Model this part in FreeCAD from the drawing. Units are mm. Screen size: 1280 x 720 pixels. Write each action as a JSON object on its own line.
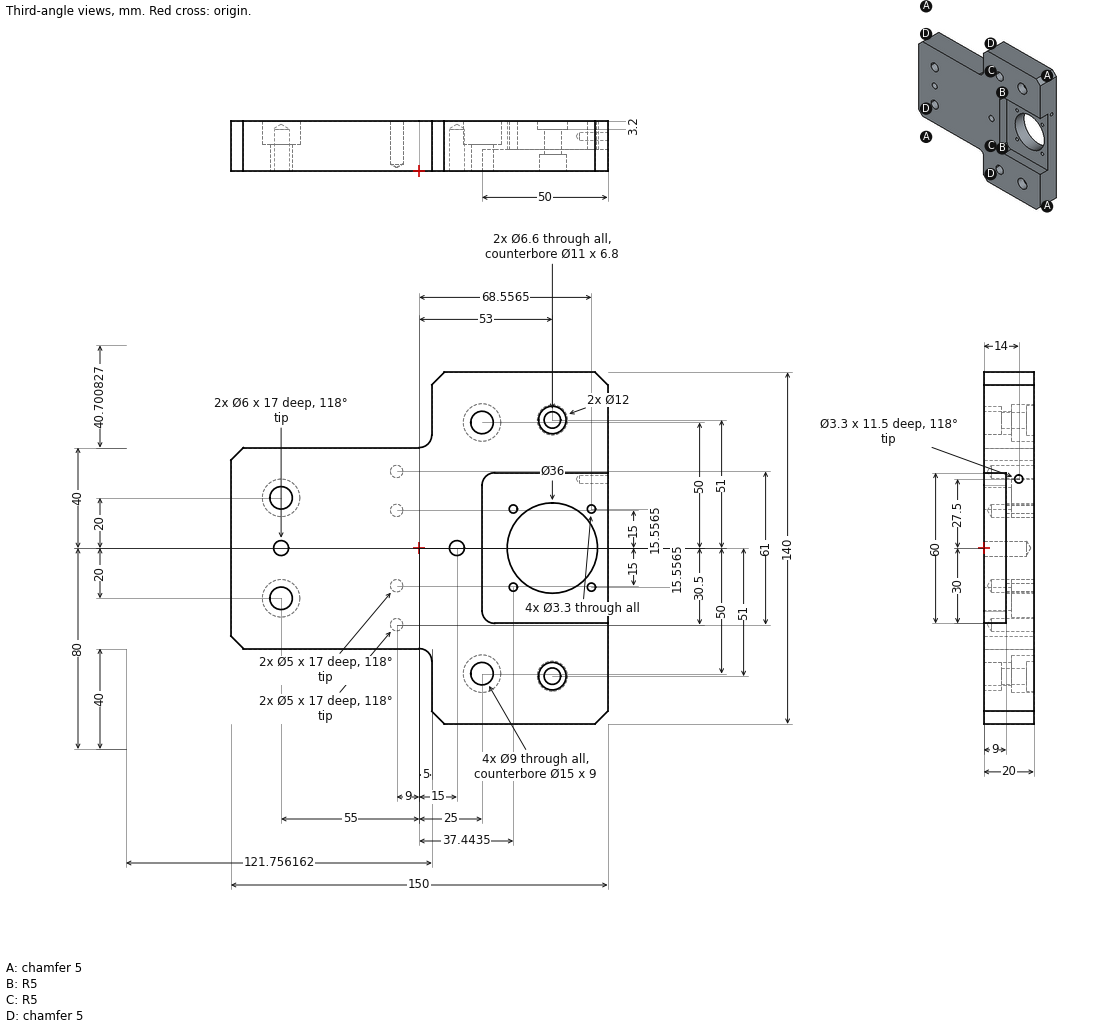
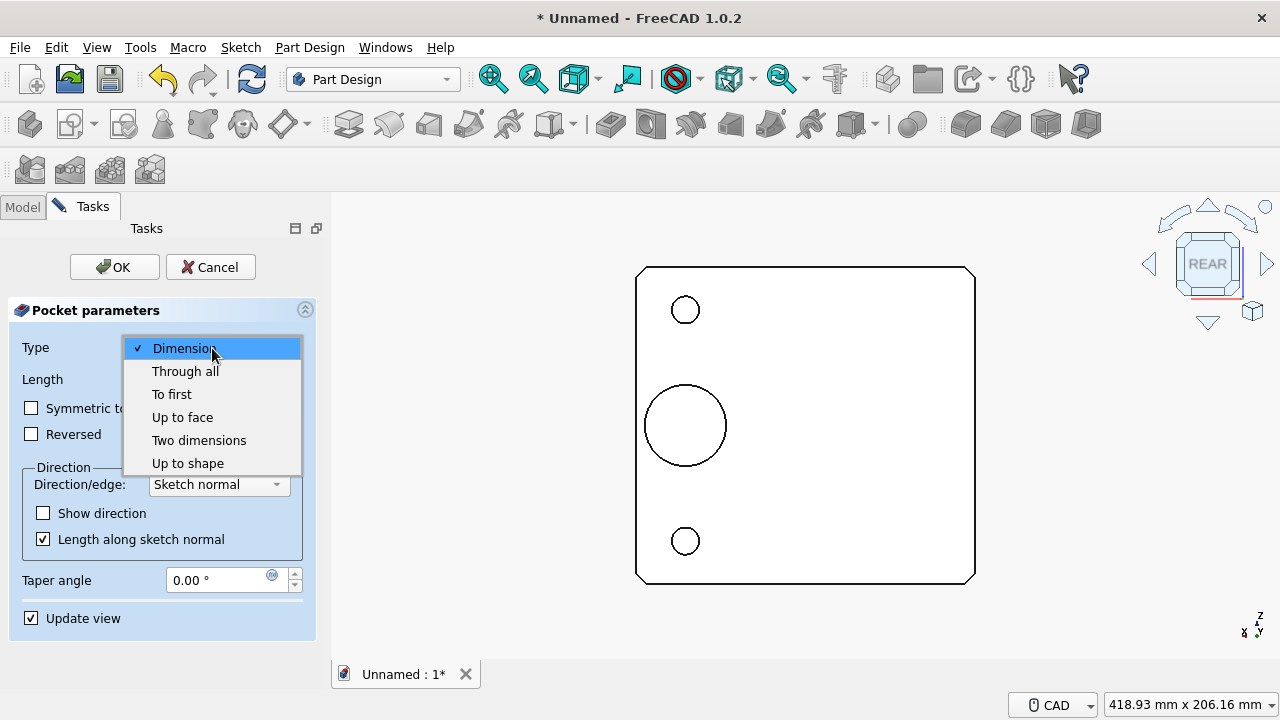
{"action": "left_click", "coordinate": [212, 372]}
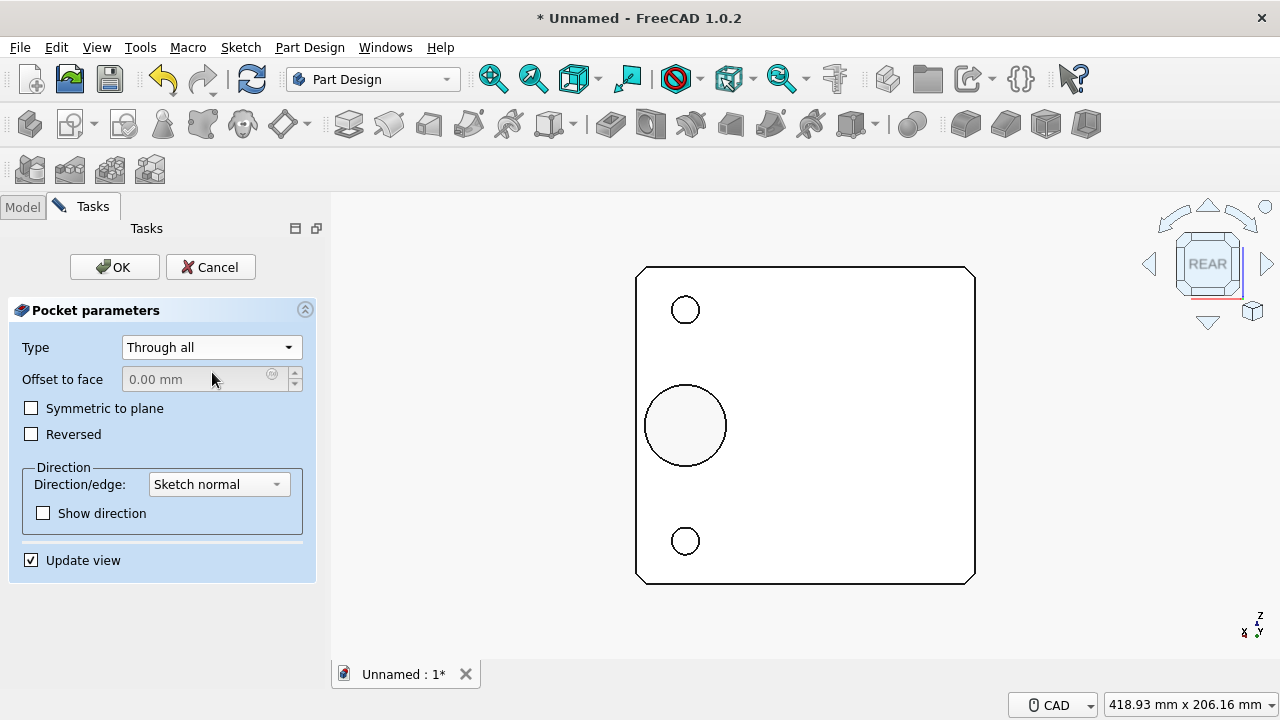
{"action": "left_click", "coordinate": [115, 267]}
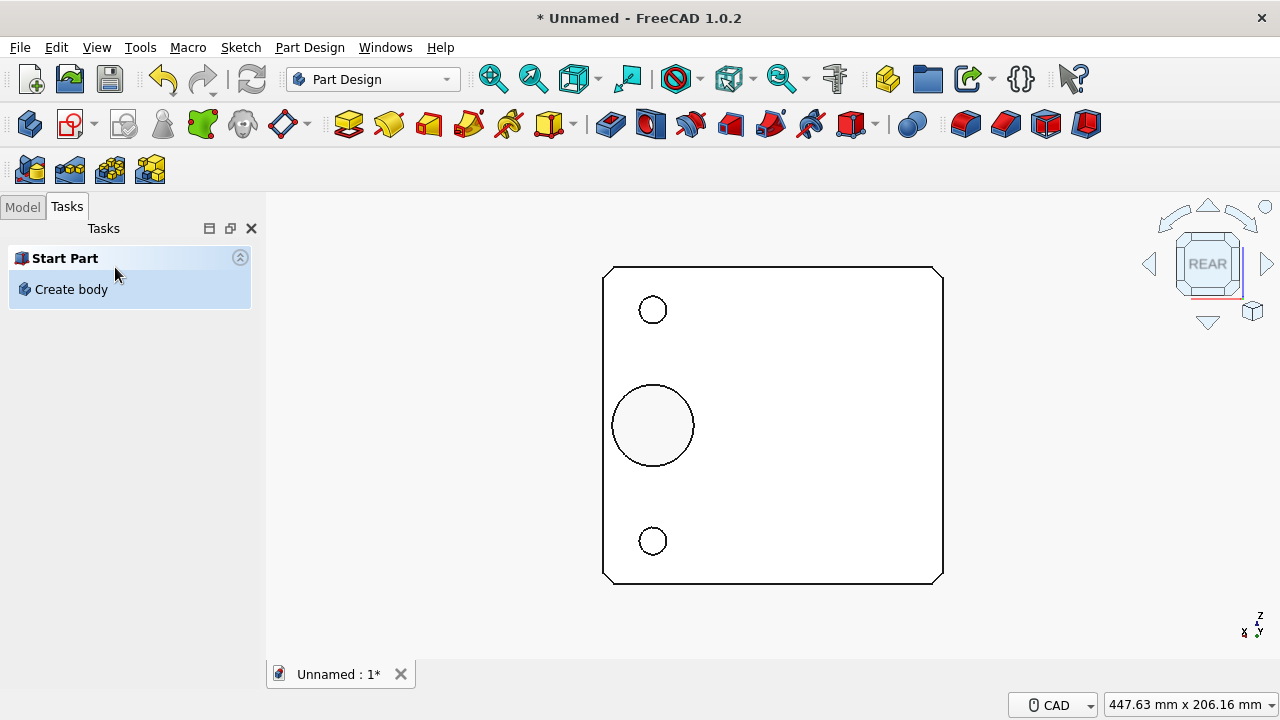
{"action": "left_click", "coordinate": [822, 424]}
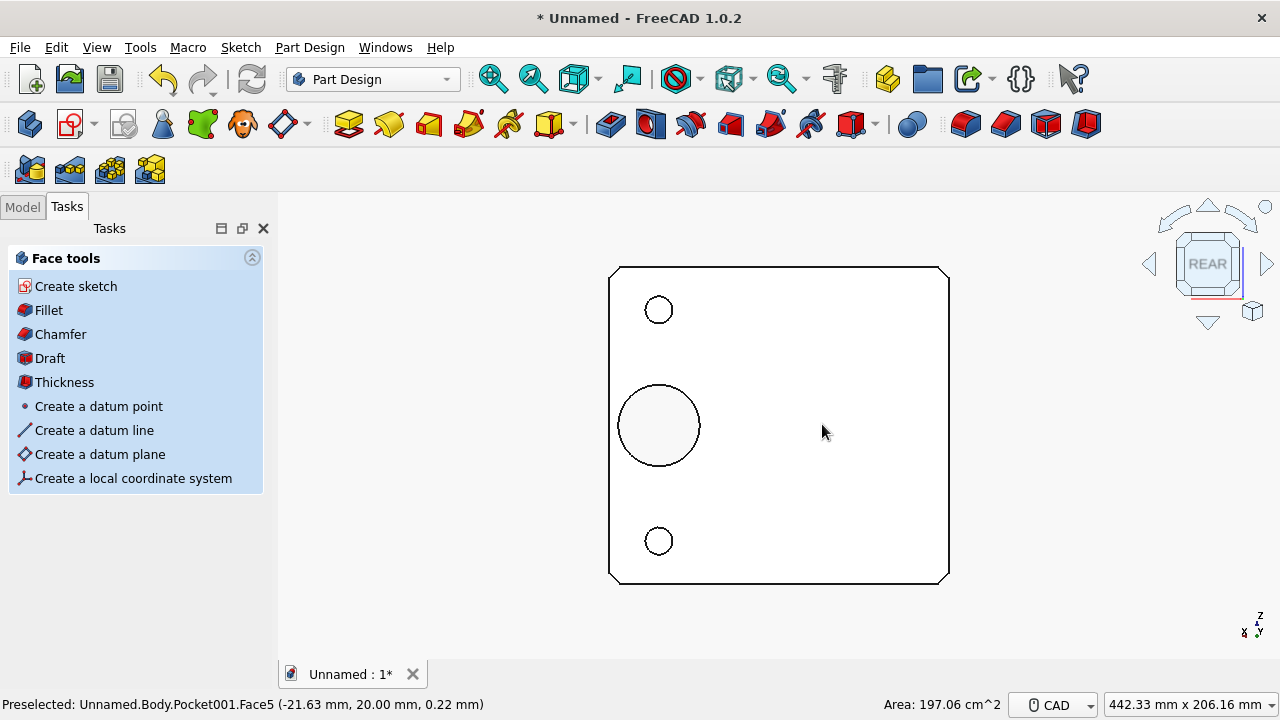
{"action": "left_click", "coordinate": [70, 124]}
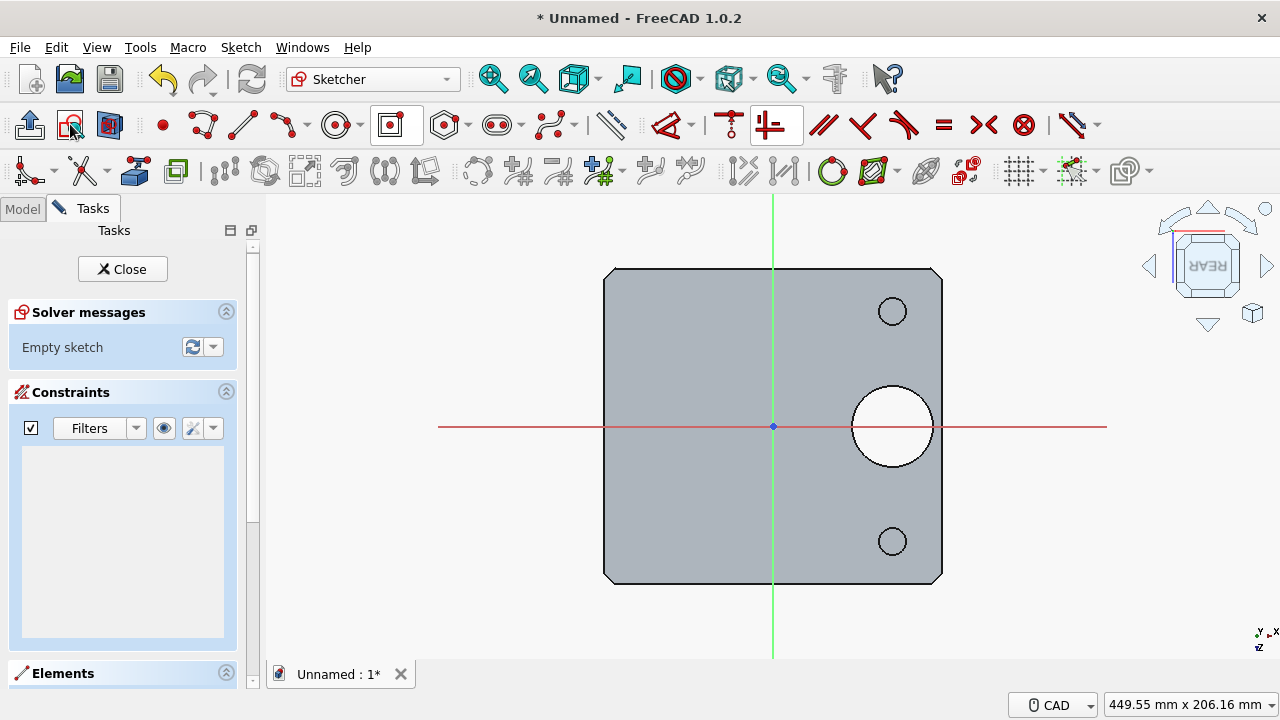
{"action": "scroll", "coordinate": [916, 426], "scroll_direction": "up", "scroll_amount": 6}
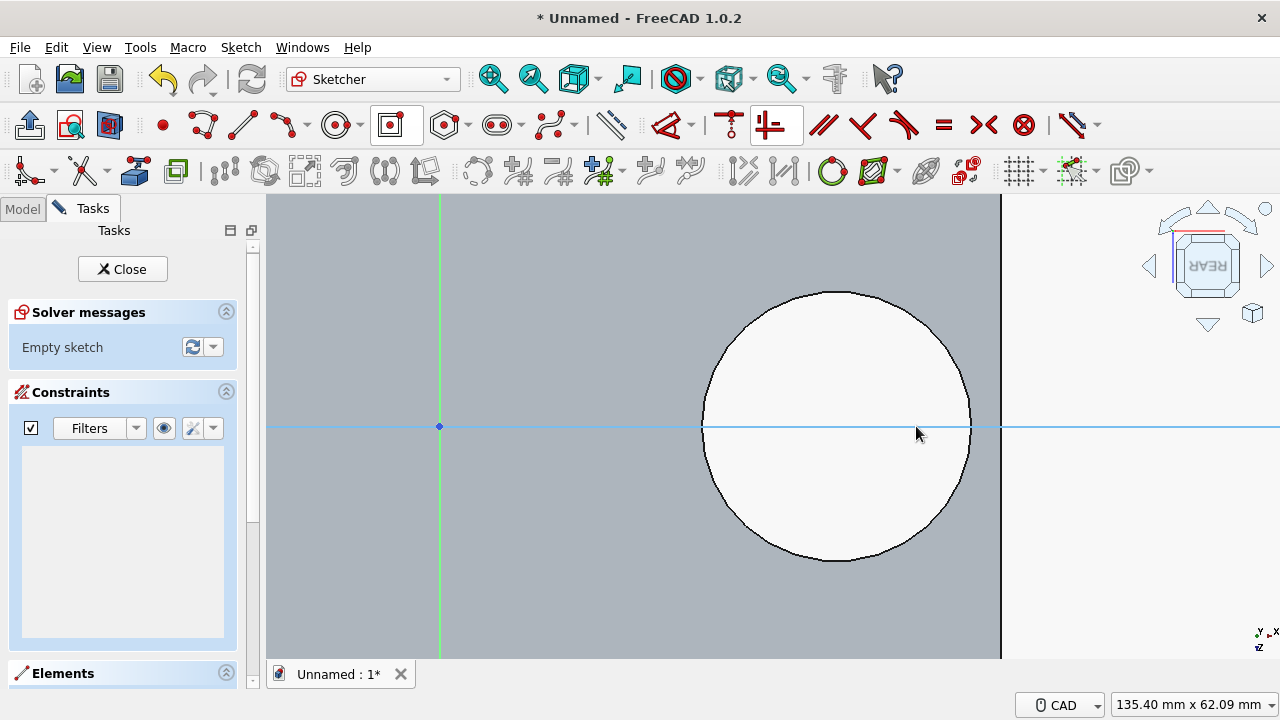
{"action": "left_click", "coordinate": [336, 126]}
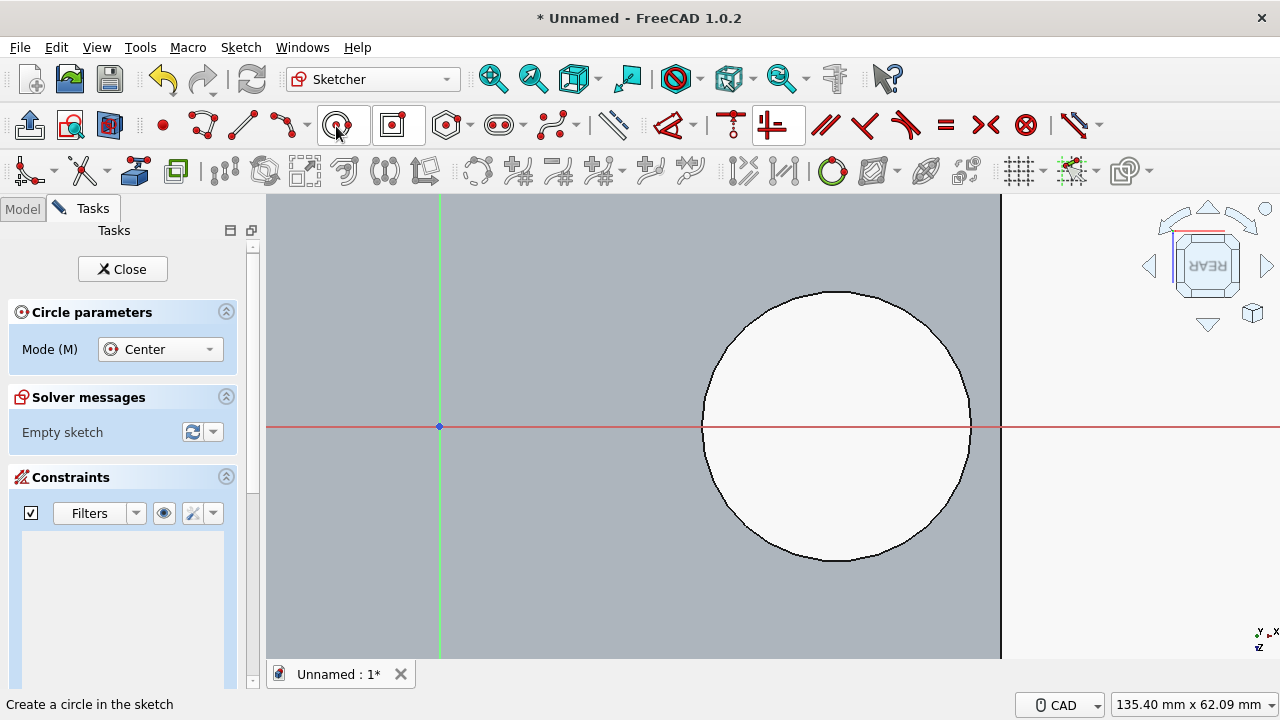
{"action": "scroll", "coordinate": [953, 543], "scroll_direction": "up", "scroll_amount": 4}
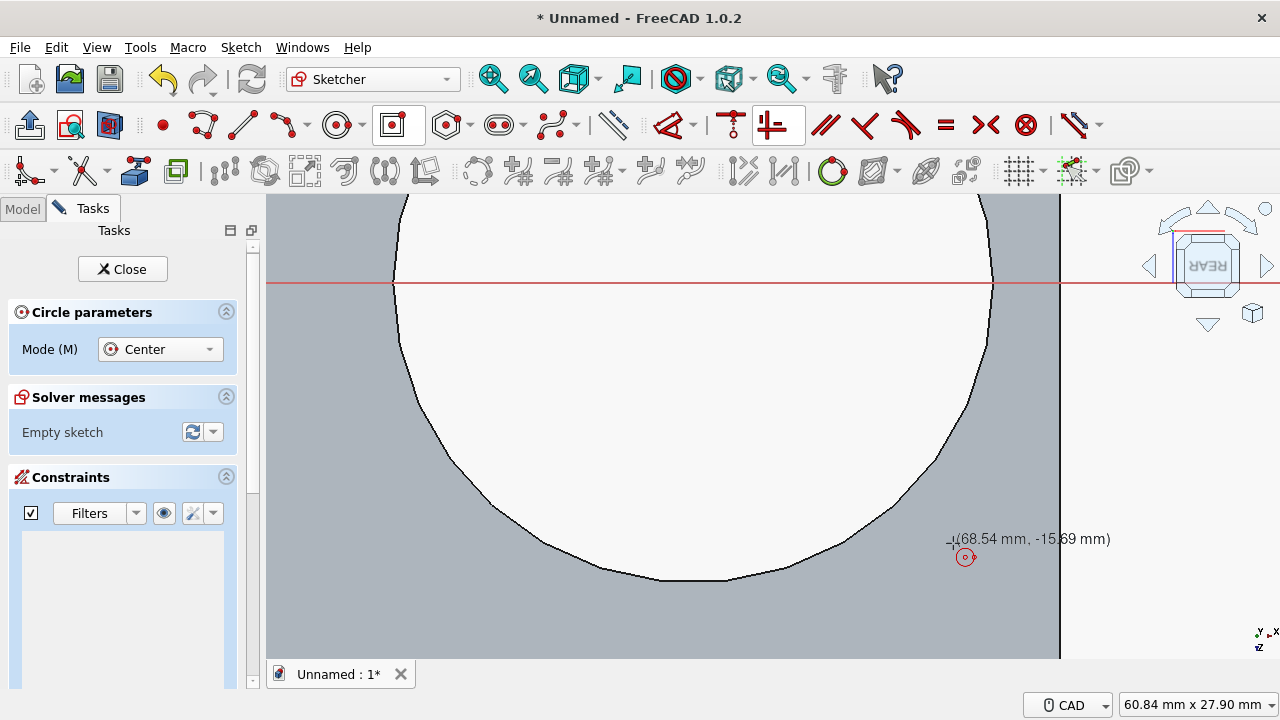
{"action": "left_click", "coordinate": [952, 542]}
{"action": "left_click", "coordinate": [972, 523]}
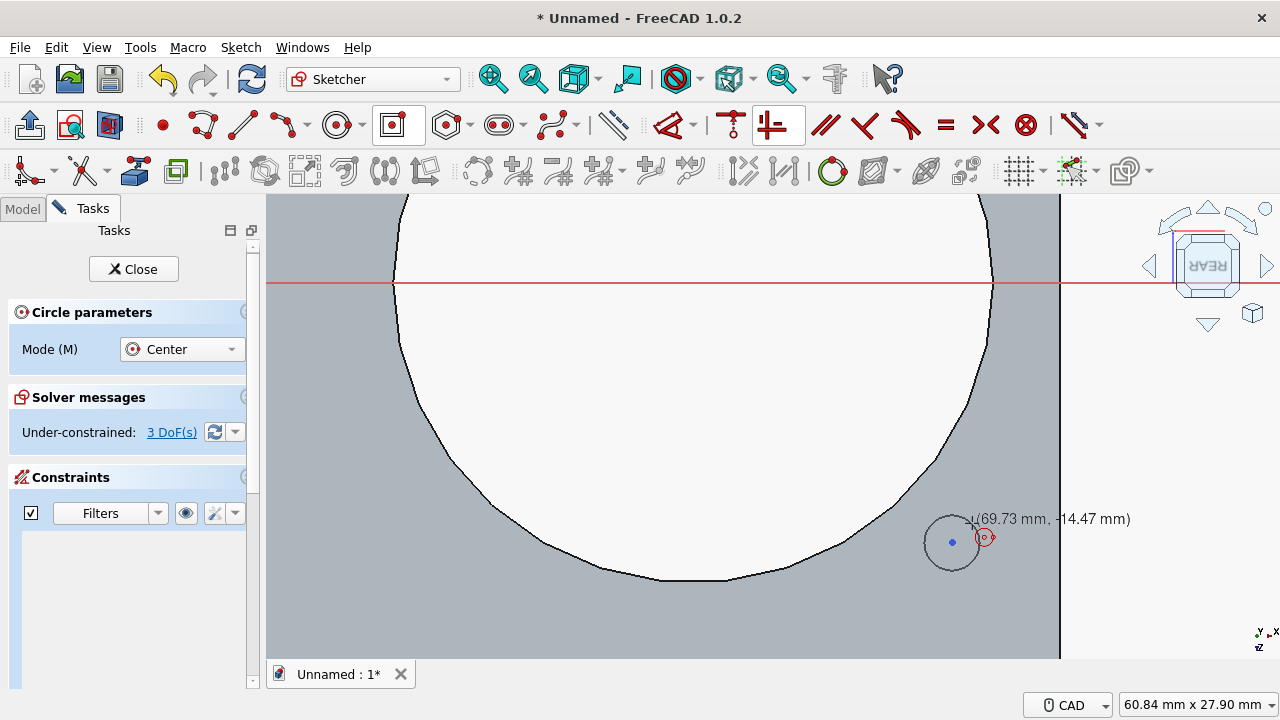
{"action": "scroll", "coordinate": [957, 544], "scroll_direction": "down", "scroll_amount": 4}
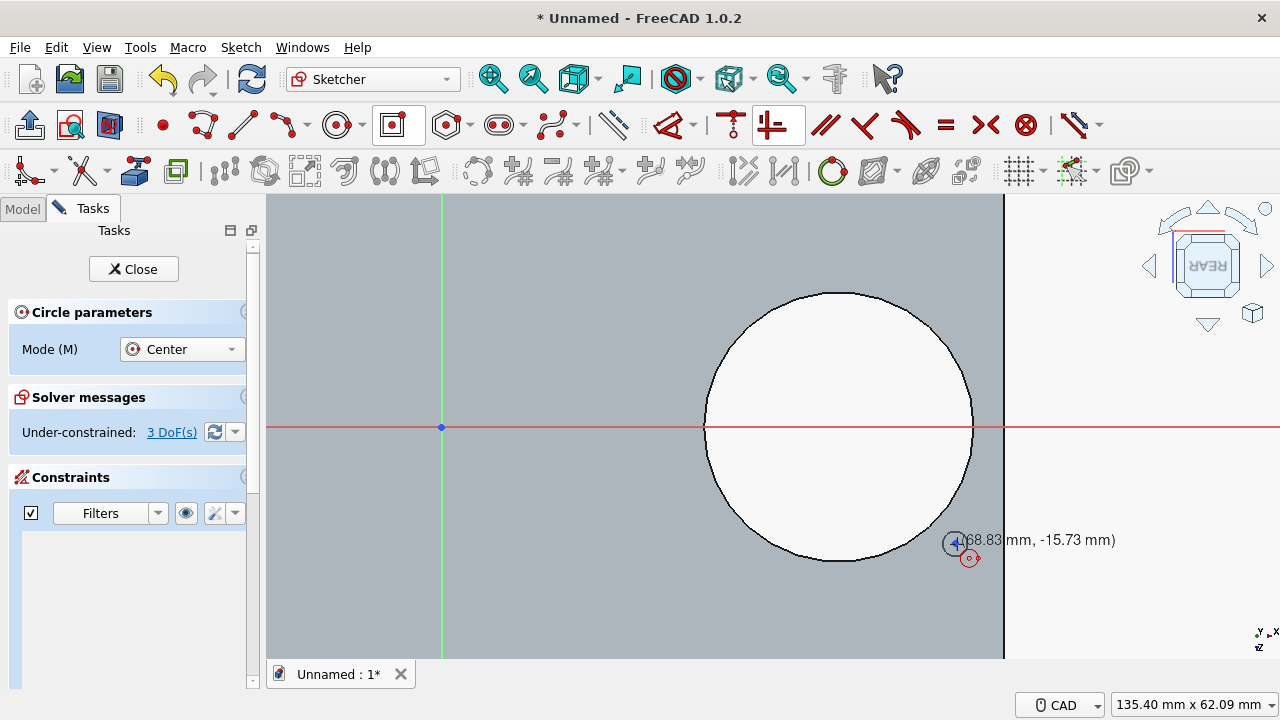
{"action": "scroll", "coordinate": [955, 311], "scroll_direction": "up", "scroll_amount": 4}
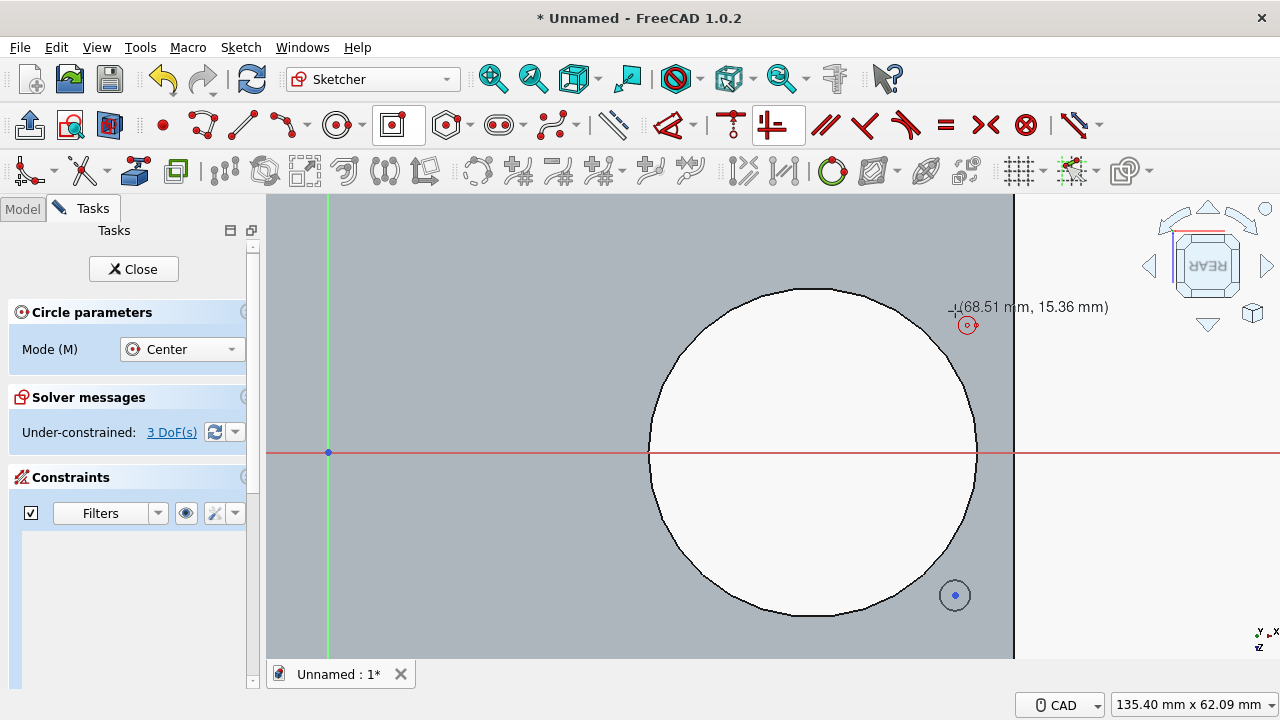
{"action": "left_click", "coordinate": [955, 310]}
{"action": "left_click", "coordinate": [974, 290]}